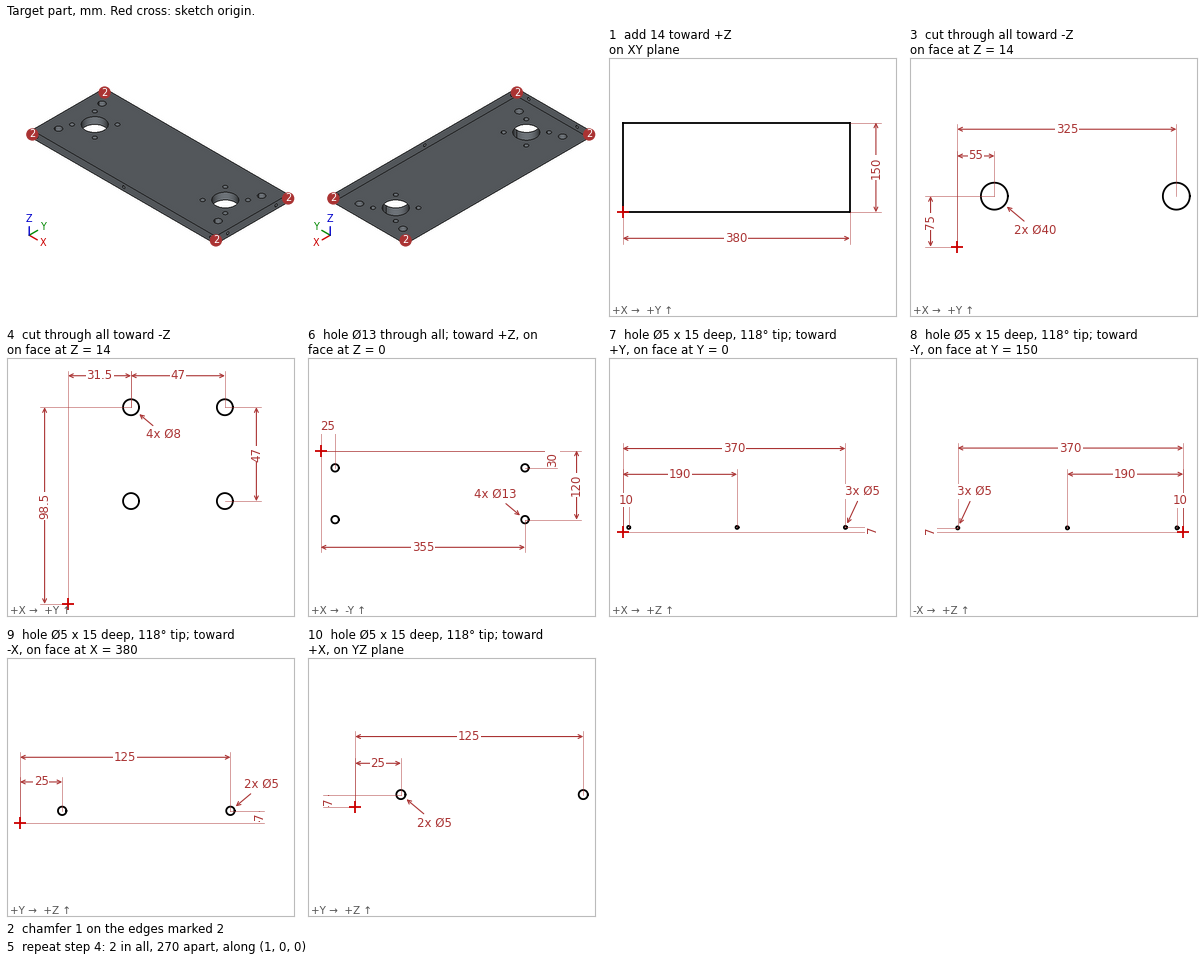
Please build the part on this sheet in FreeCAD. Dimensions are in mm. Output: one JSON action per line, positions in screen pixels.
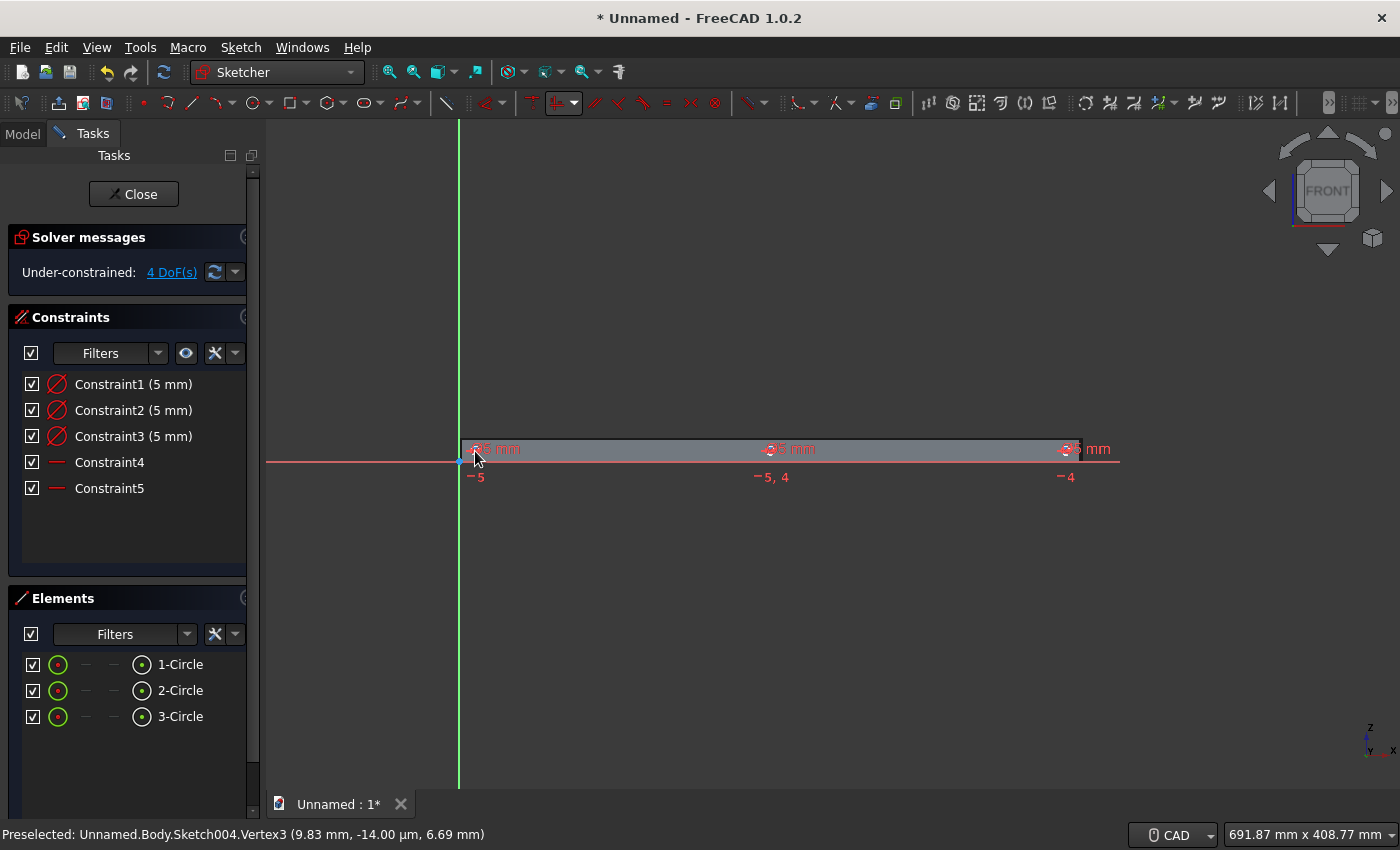
{"action": "left_click", "coordinate": [486, 104]}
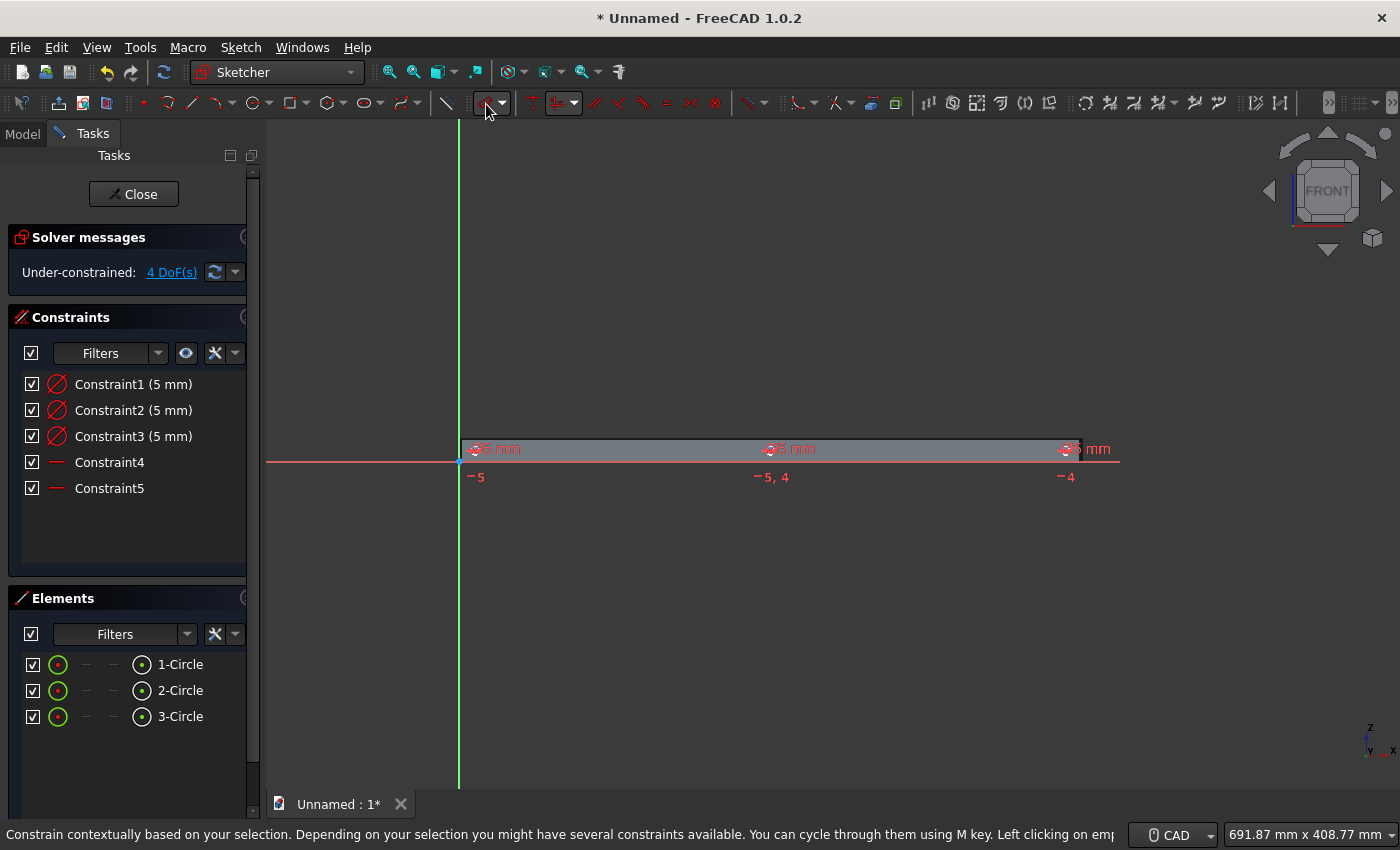
{"action": "scroll", "coordinate": [1066, 451], "scroll_direction": "up", "scroll_amount": 7}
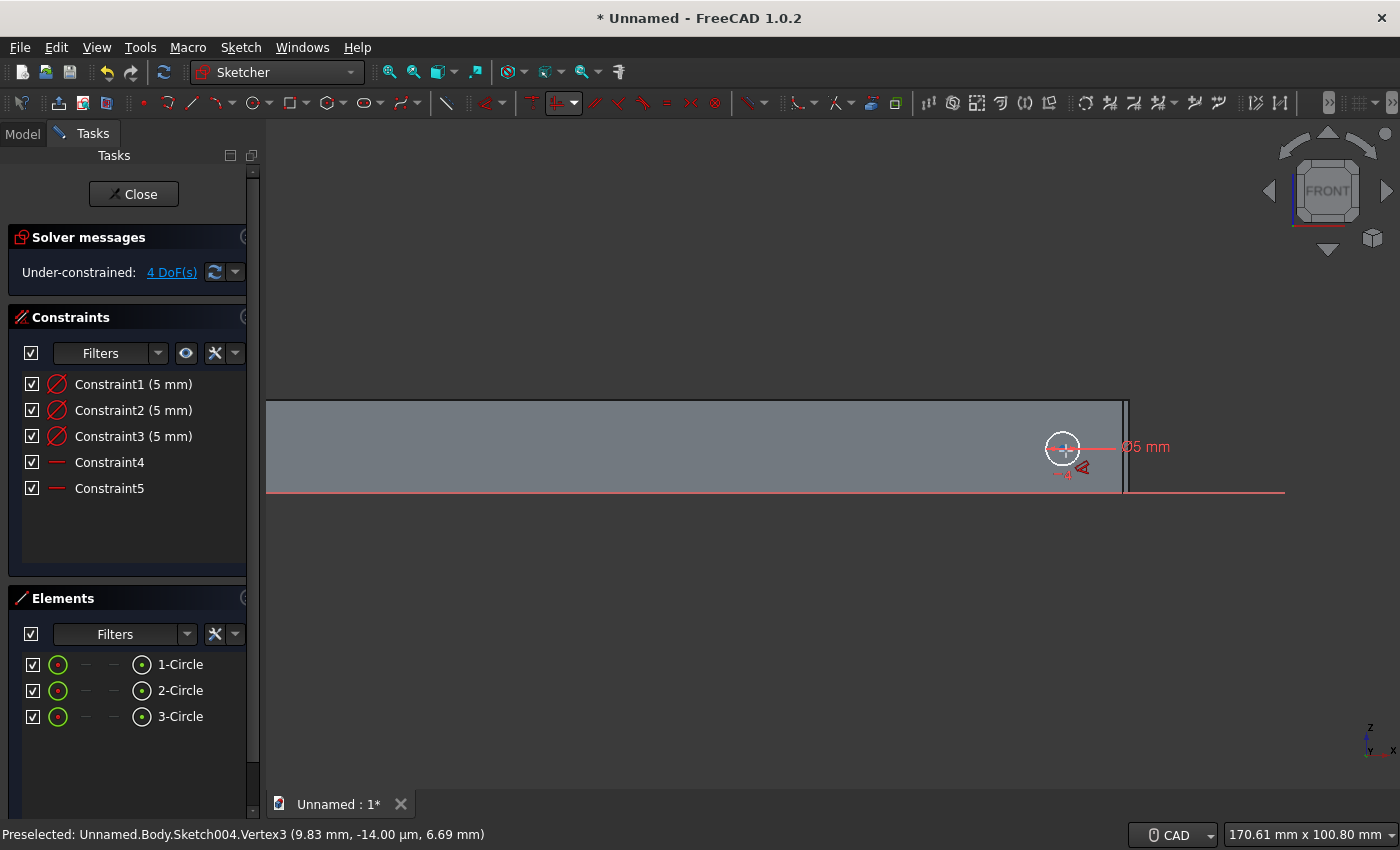
{"action": "left_click", "coordinate": [1063, 449]}
{"action": "left_click", "coordinate": [1097, 471]}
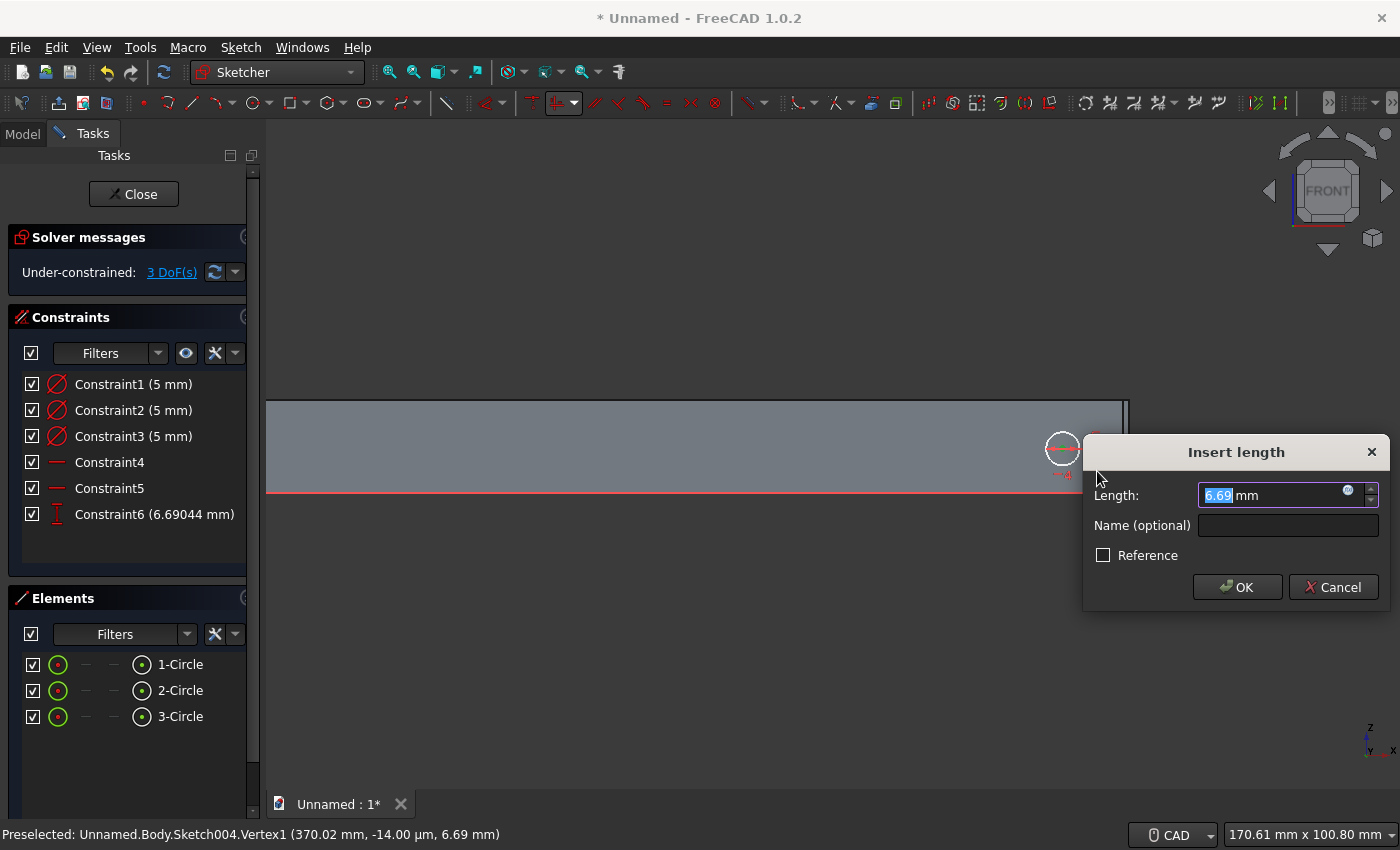
{"action": "type", "text": "7"}
{"action": "key", "text": "Return"}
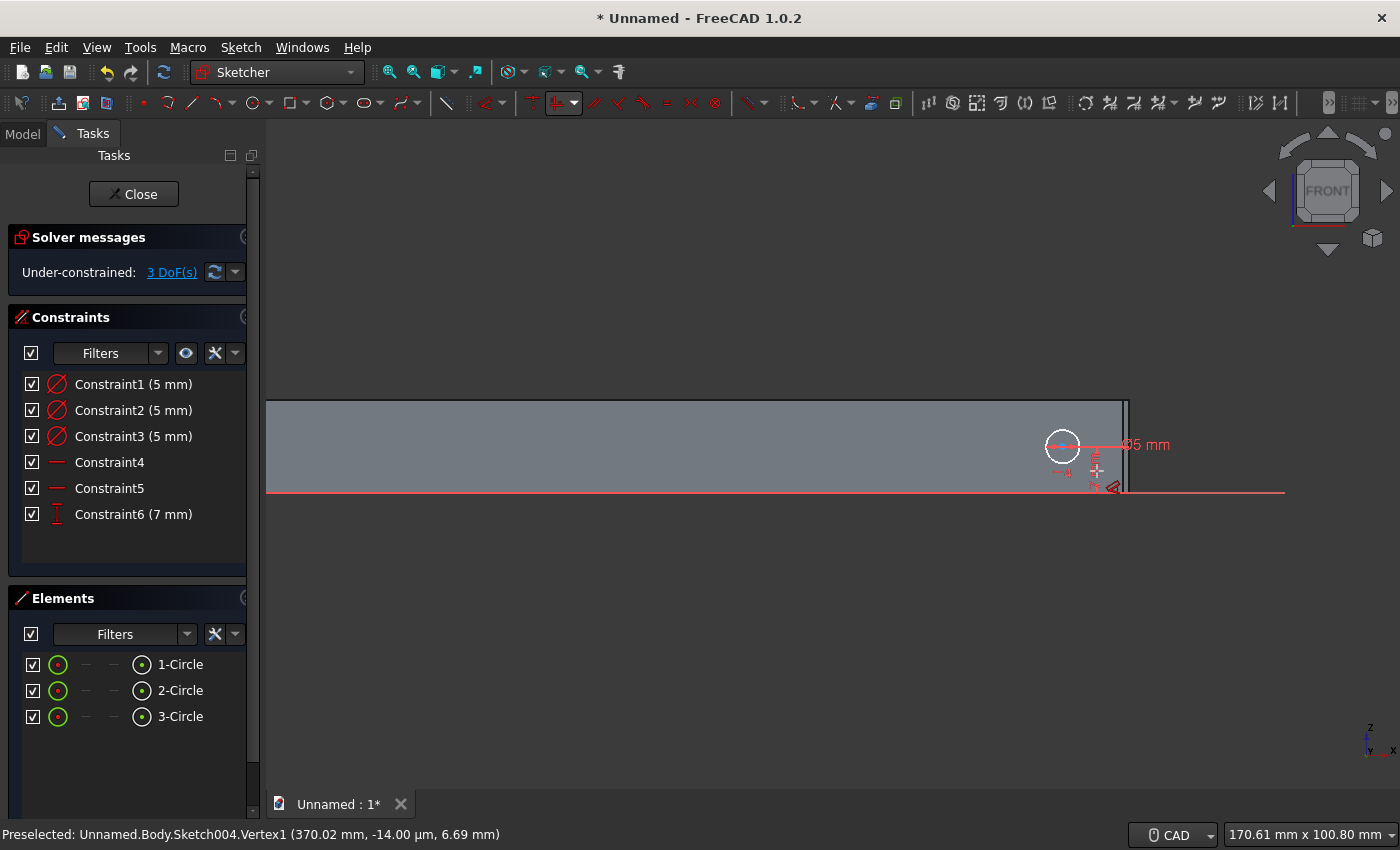
{"action": "scroll", "coordinate": [1067, 451], "scroll_direction": "down", "scroll_amount": 7}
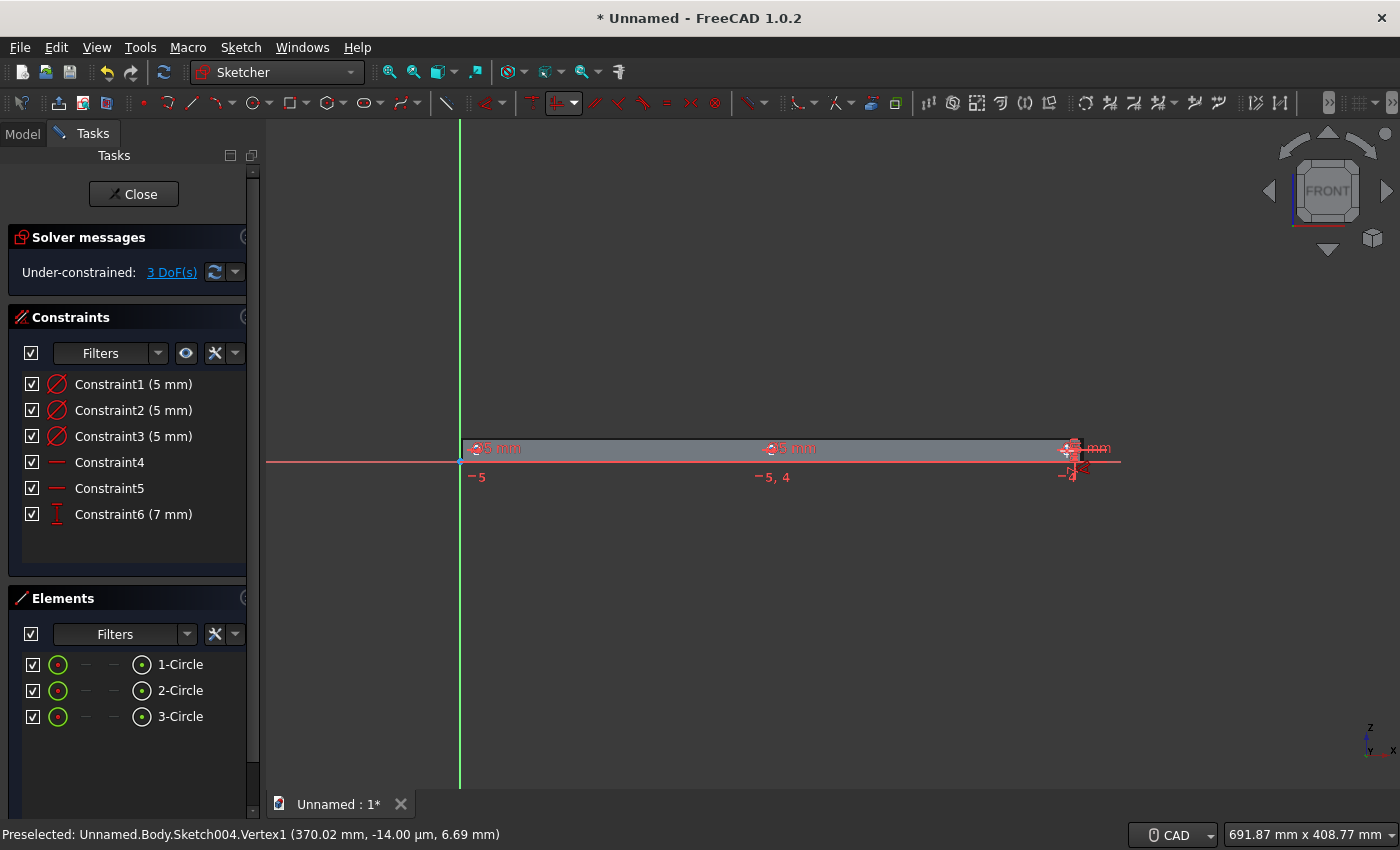
{"action": "scroll", "coordinate": [476, 450], "scroll_direction": "up", "scroll_amount": 5}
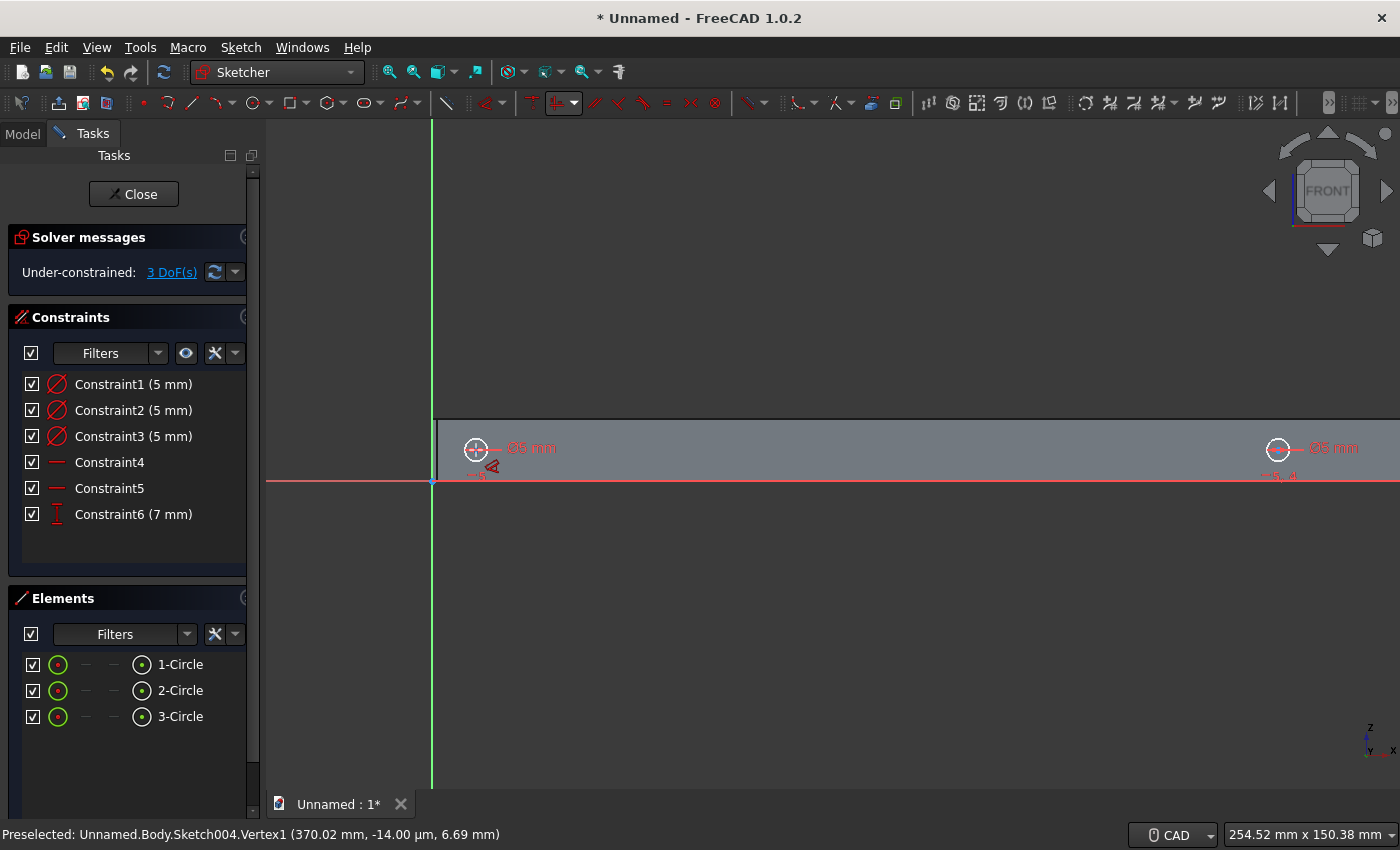
{"action": "left_click", "coordinate": [476, 450]}
{"action": "left_click", "coordinate": [454, 515]}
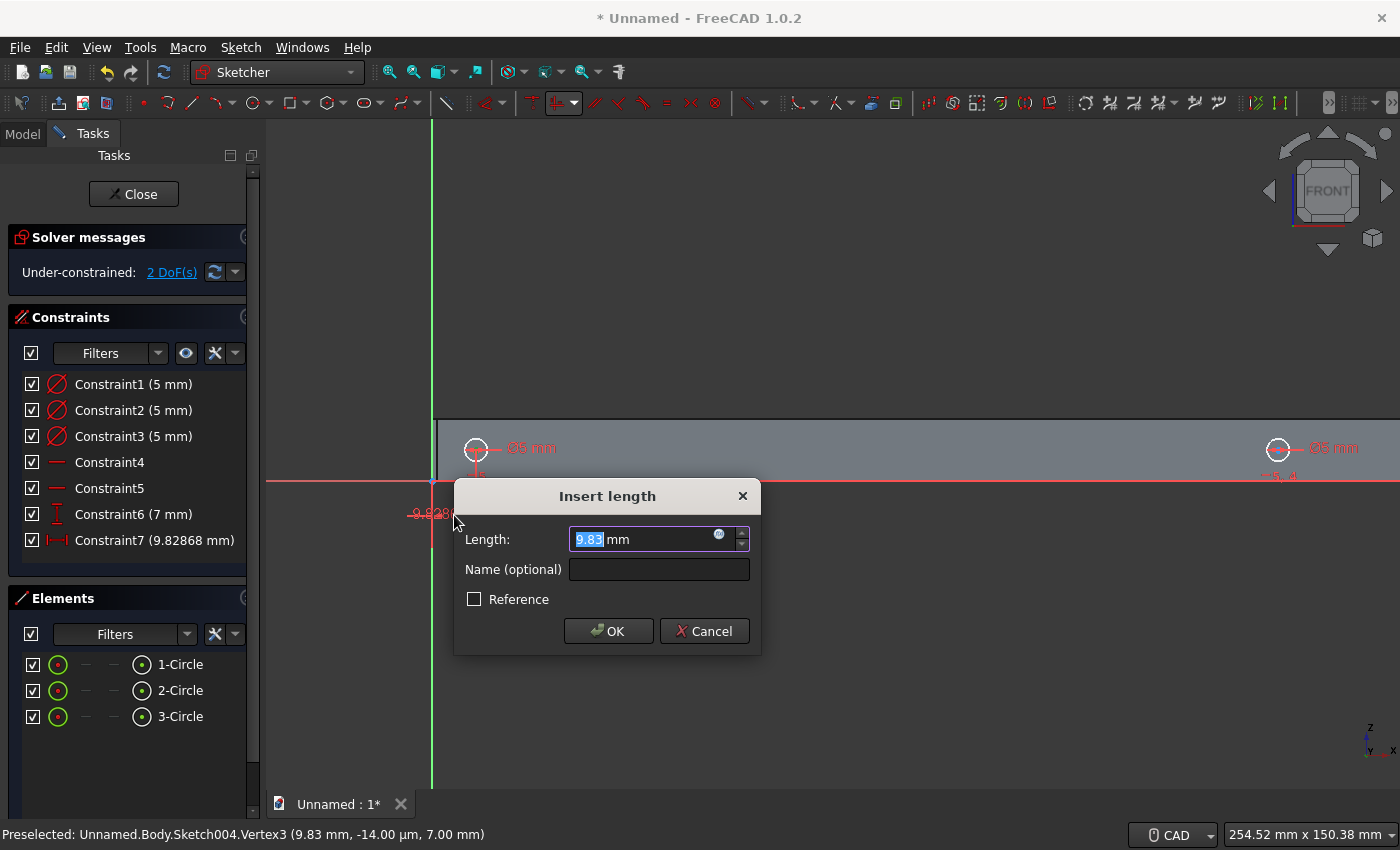
{"action": "type", "text": "10"}
{"action": "key", "text": "Return"}